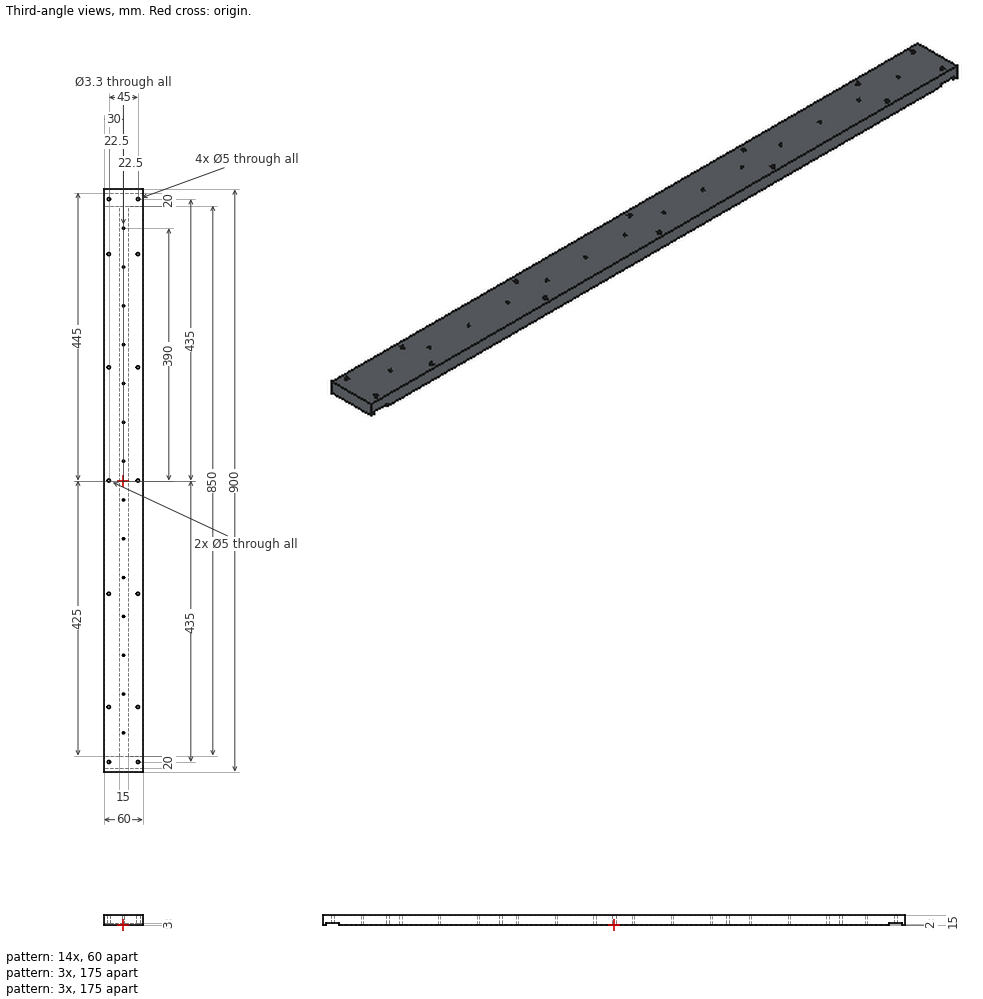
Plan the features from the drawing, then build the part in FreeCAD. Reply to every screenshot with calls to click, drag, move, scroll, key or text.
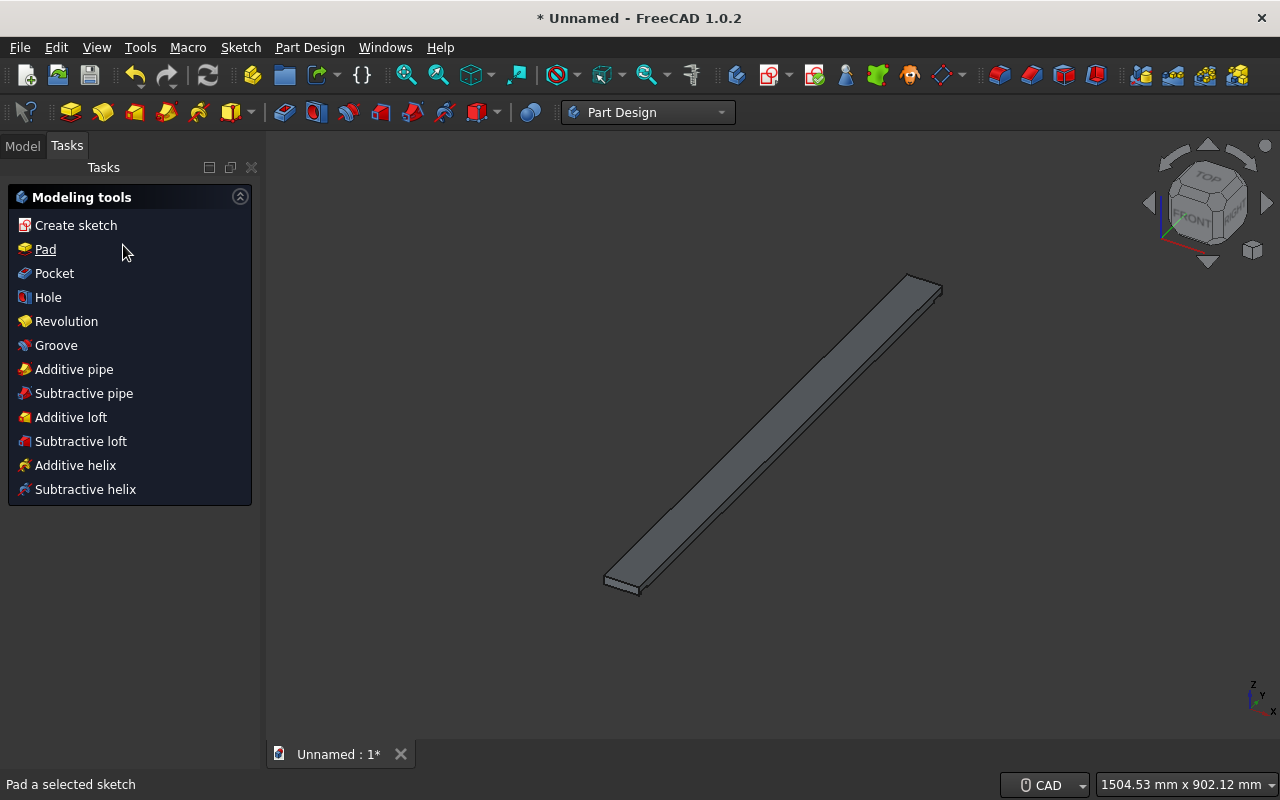
click(286, 112)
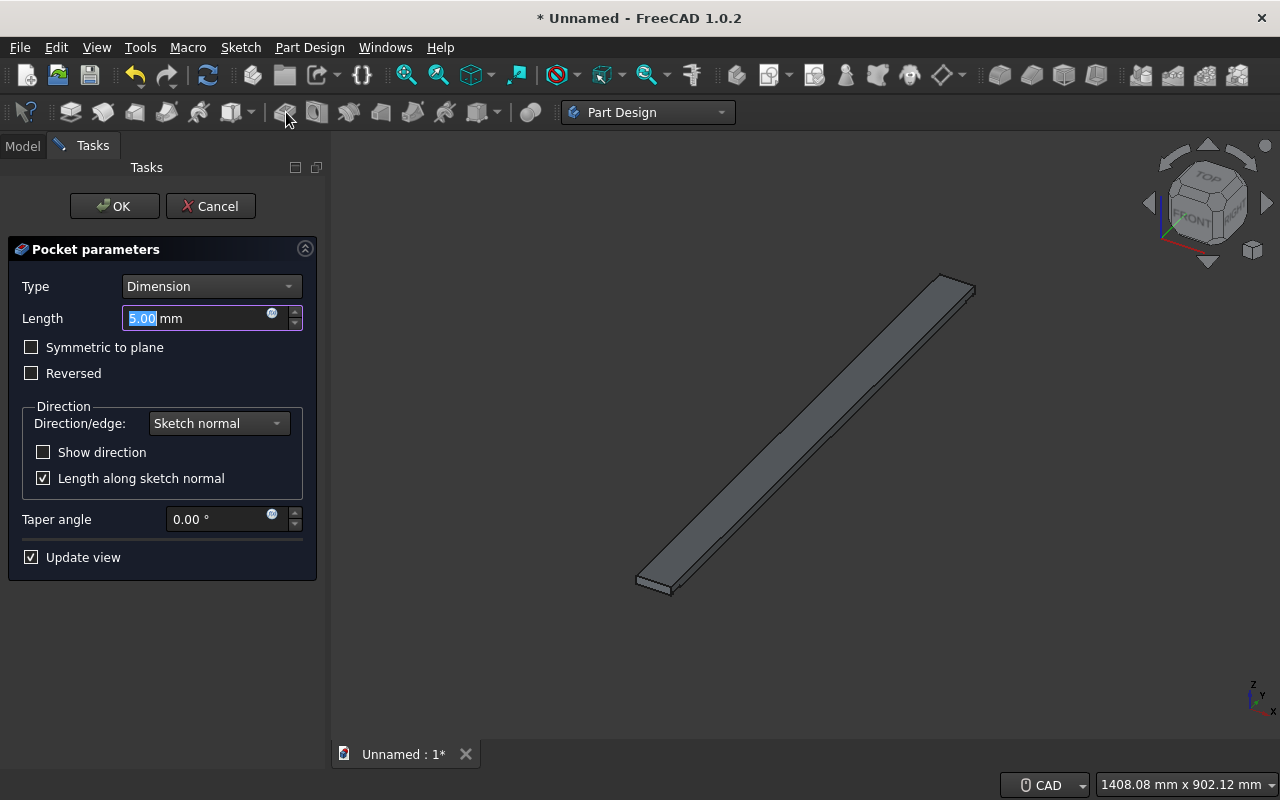
text(2)
key(Tab)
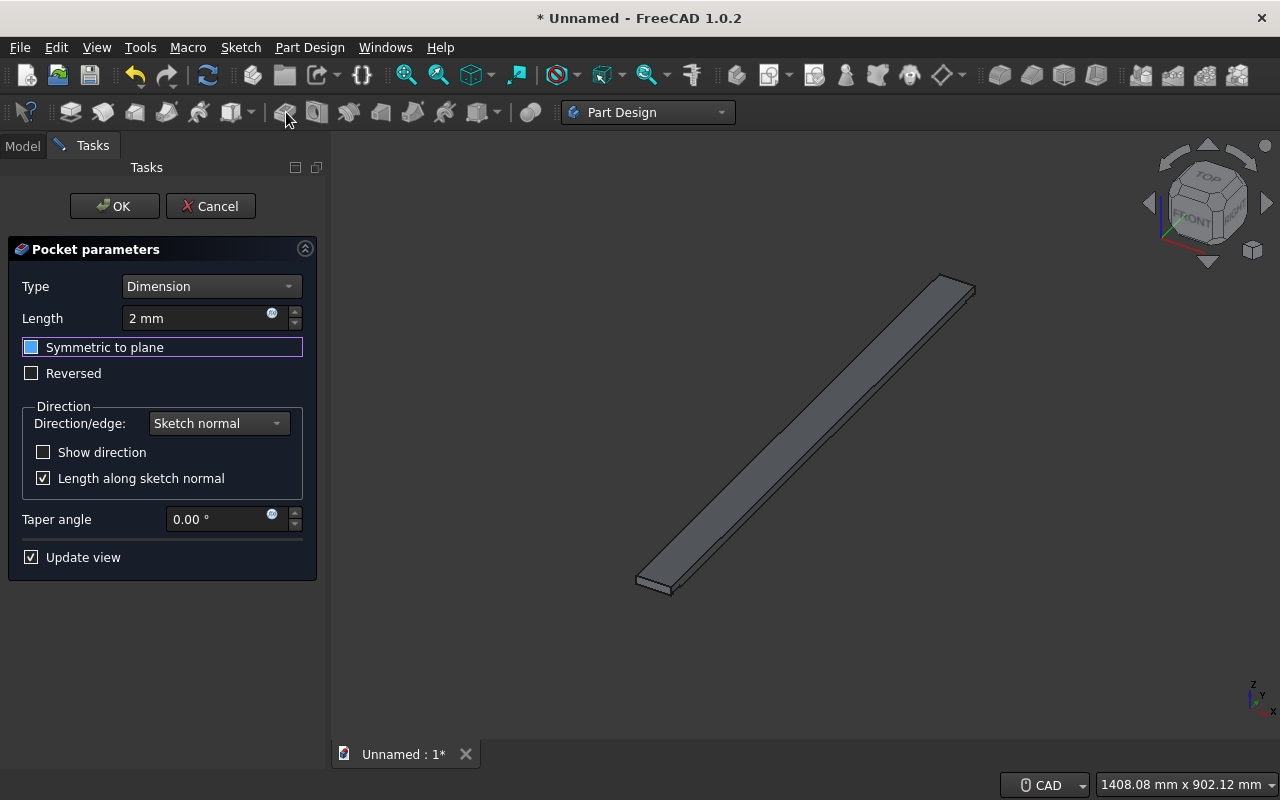
click(30, 373)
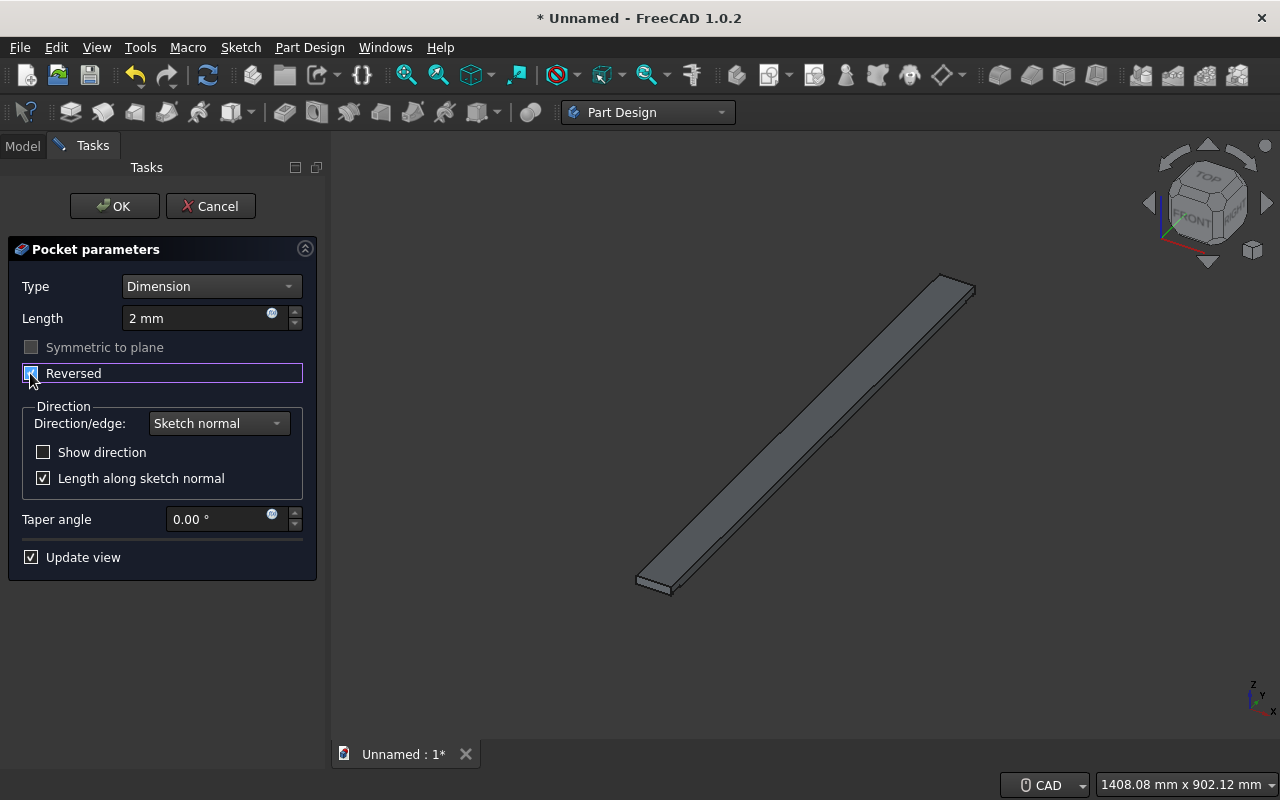
click(115, 206)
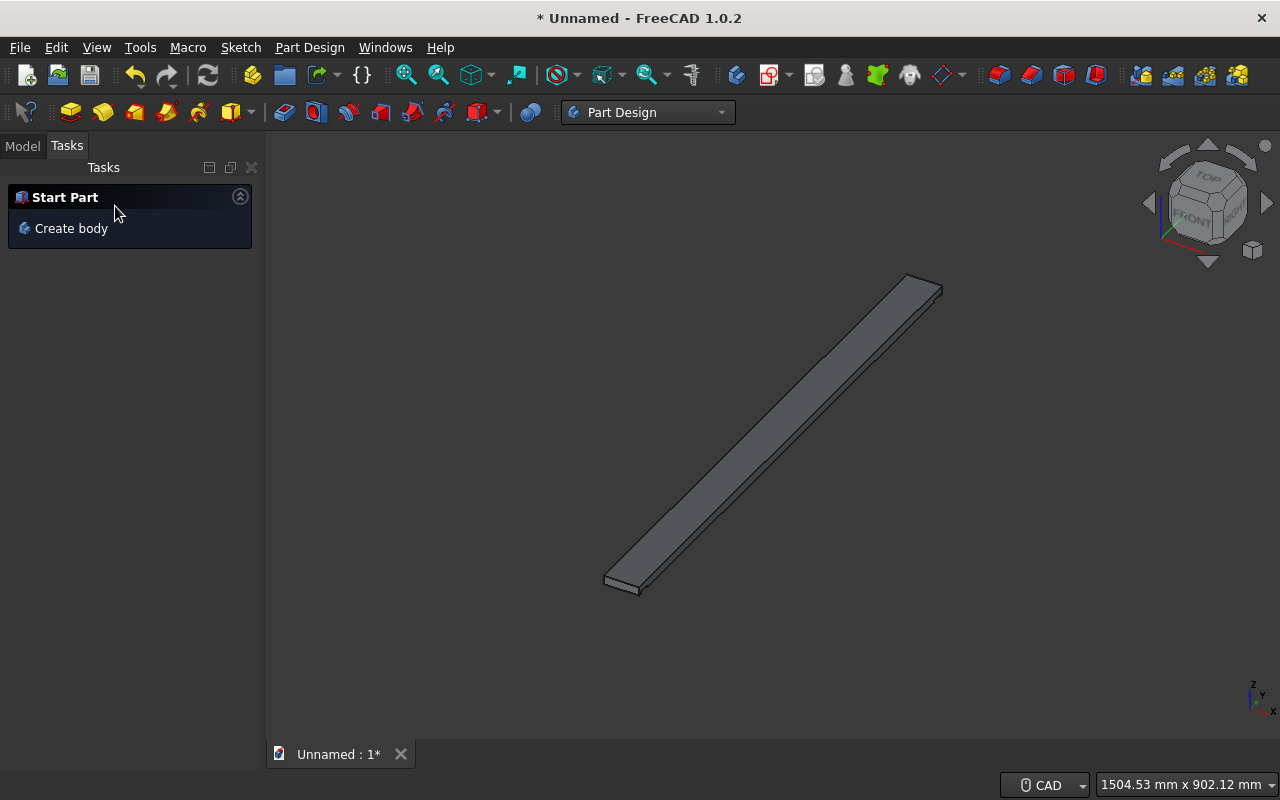
key(5)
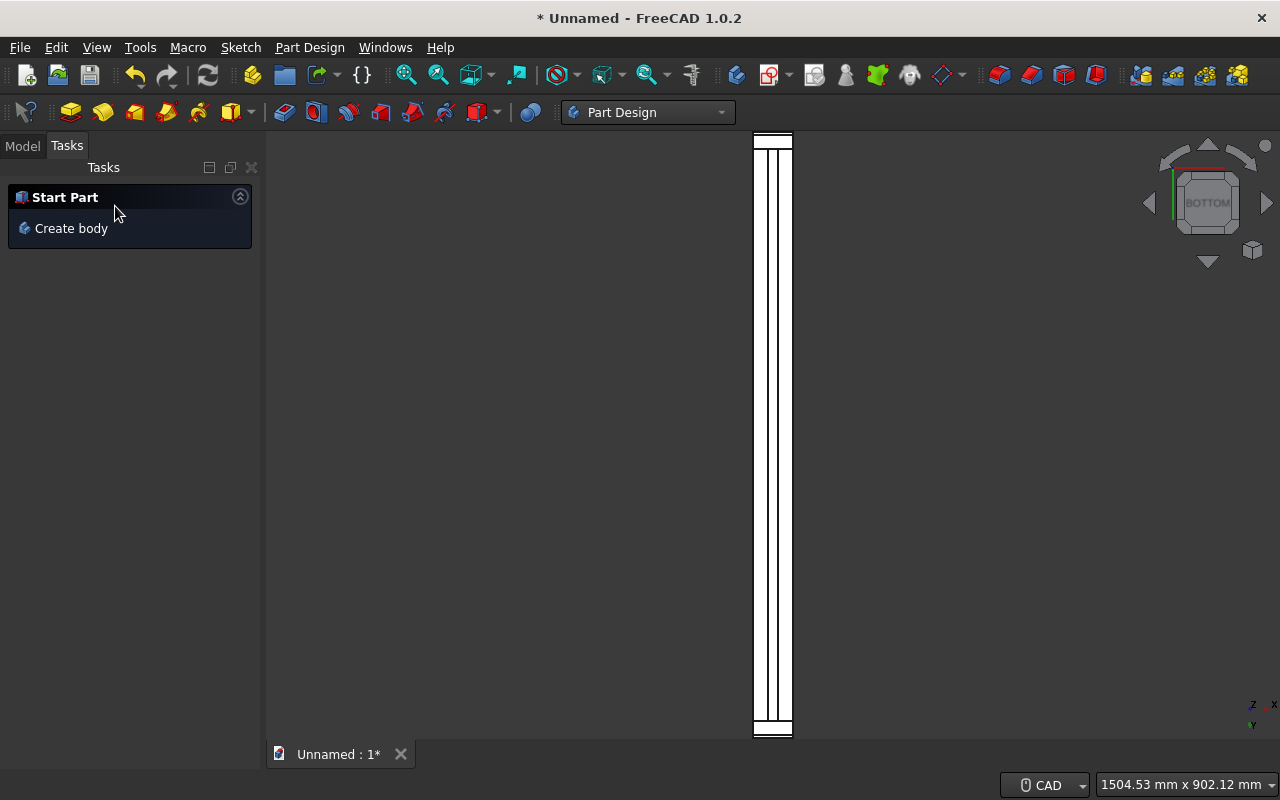
scroll(773, 680, up, 5)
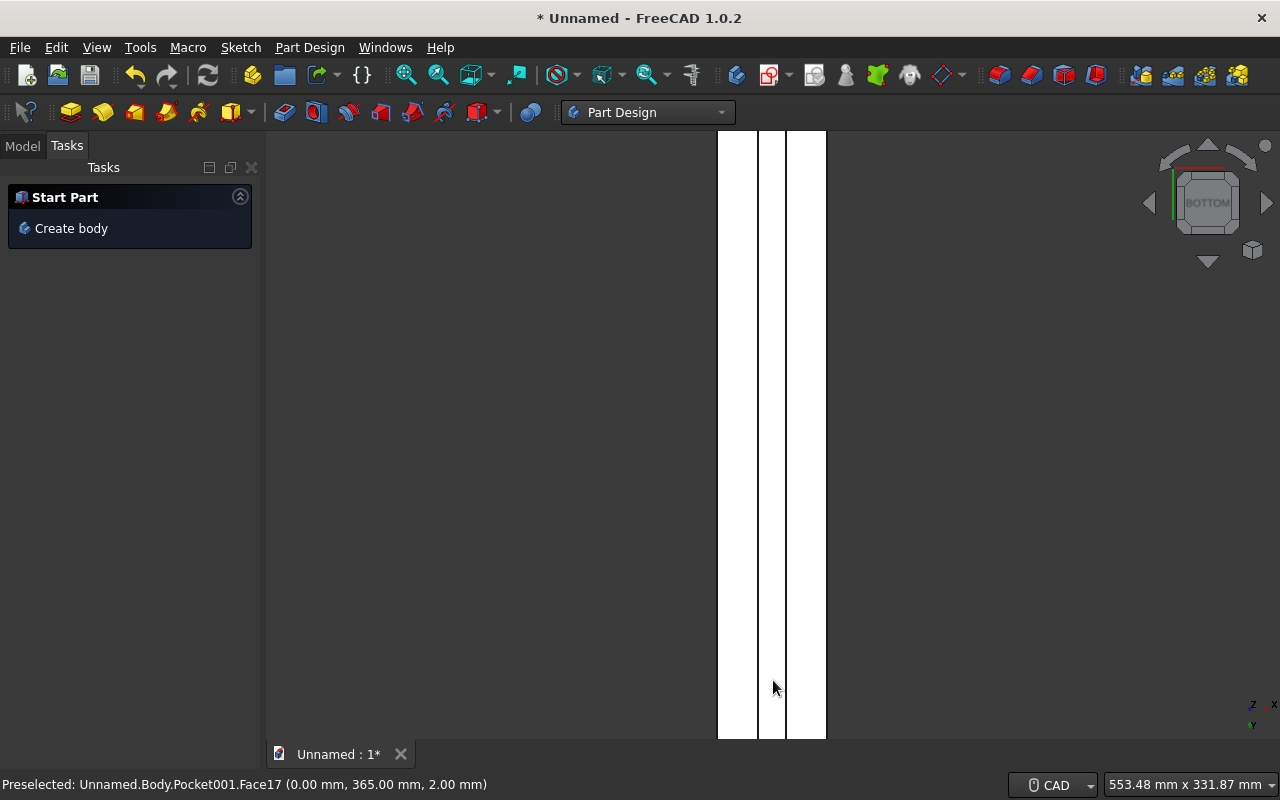
click(772, 679)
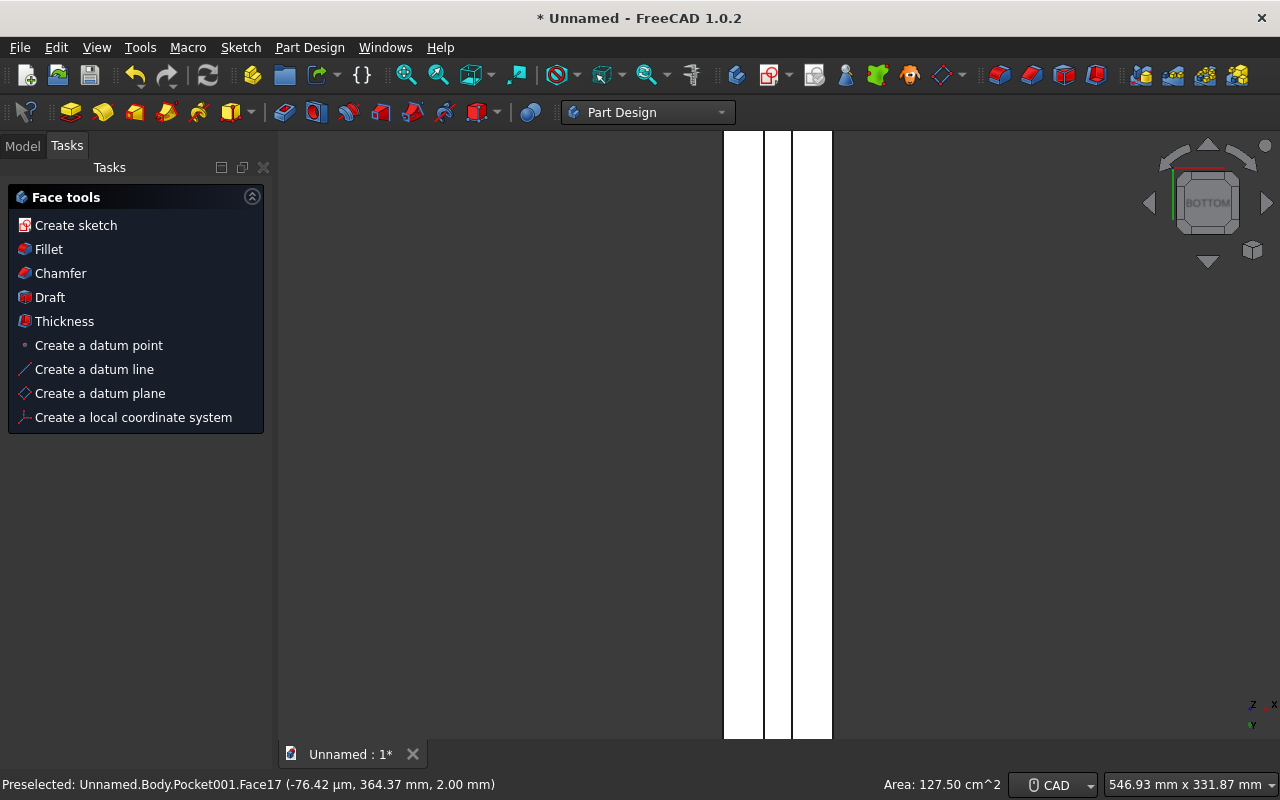
click(770, 76)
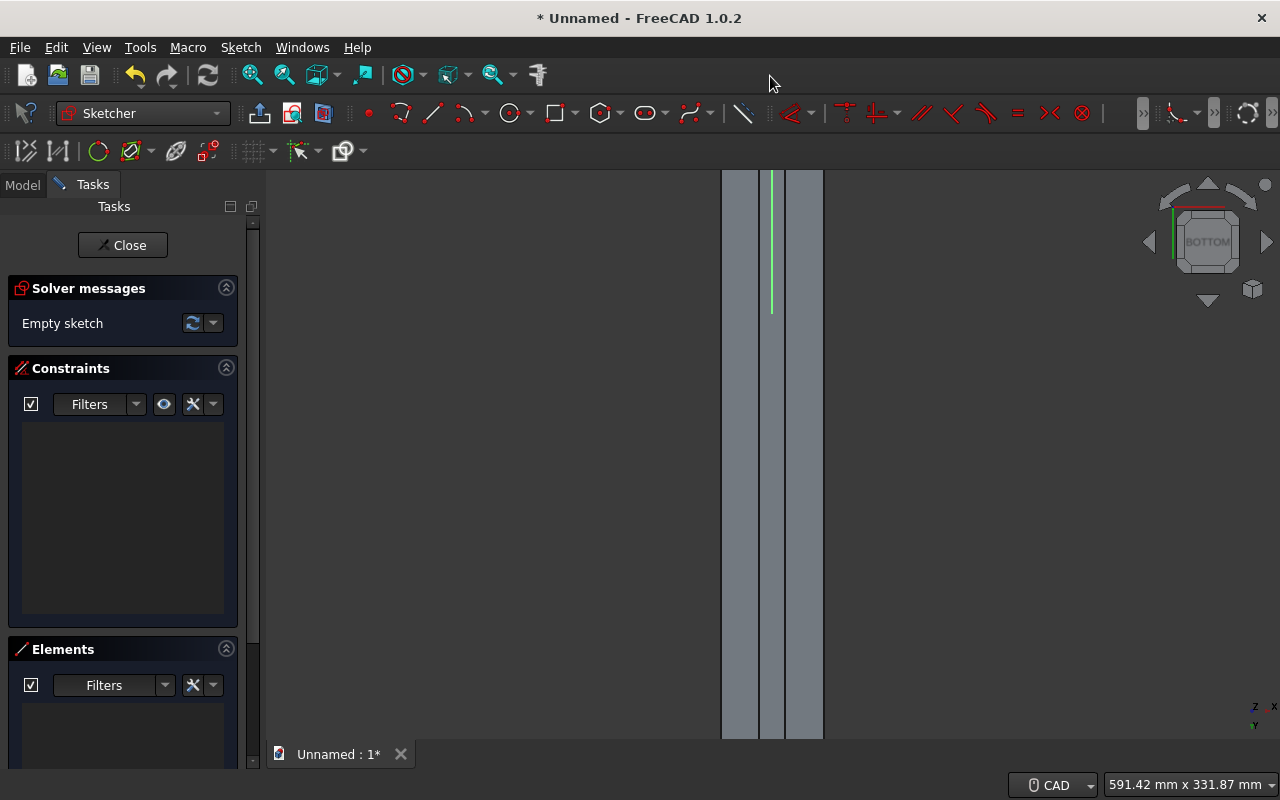
click(324, 114)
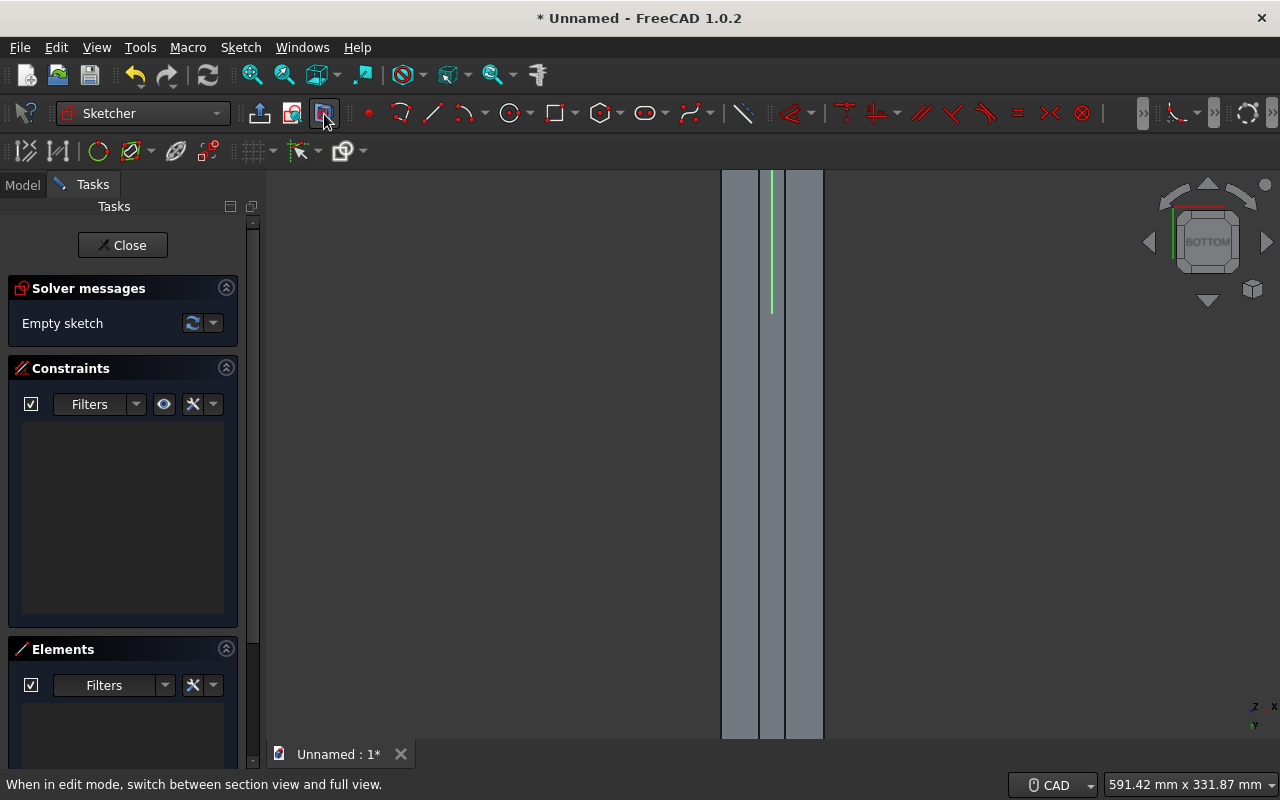
scroll(704, 454, down, 5)